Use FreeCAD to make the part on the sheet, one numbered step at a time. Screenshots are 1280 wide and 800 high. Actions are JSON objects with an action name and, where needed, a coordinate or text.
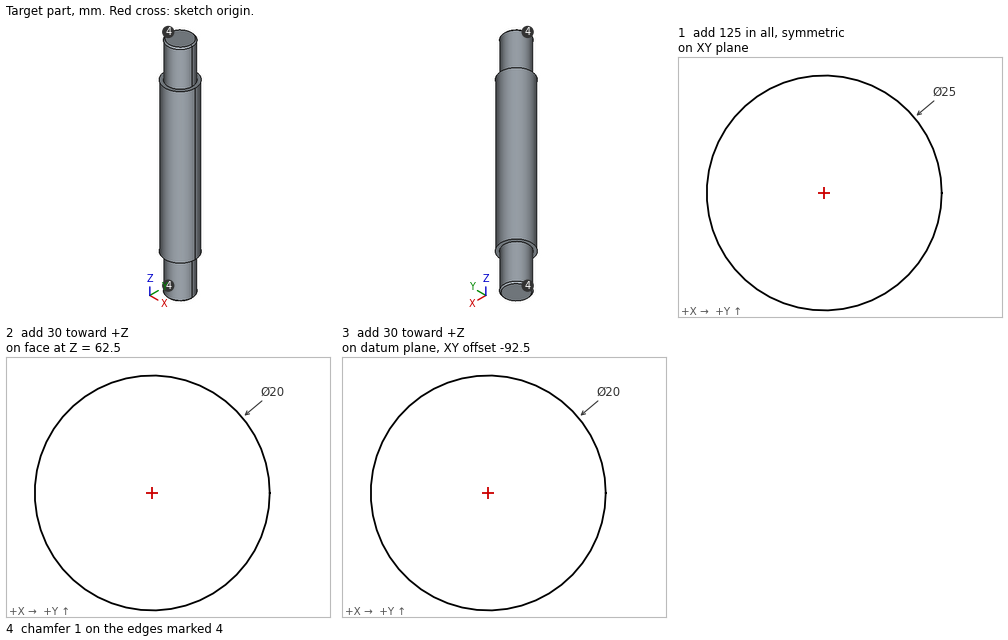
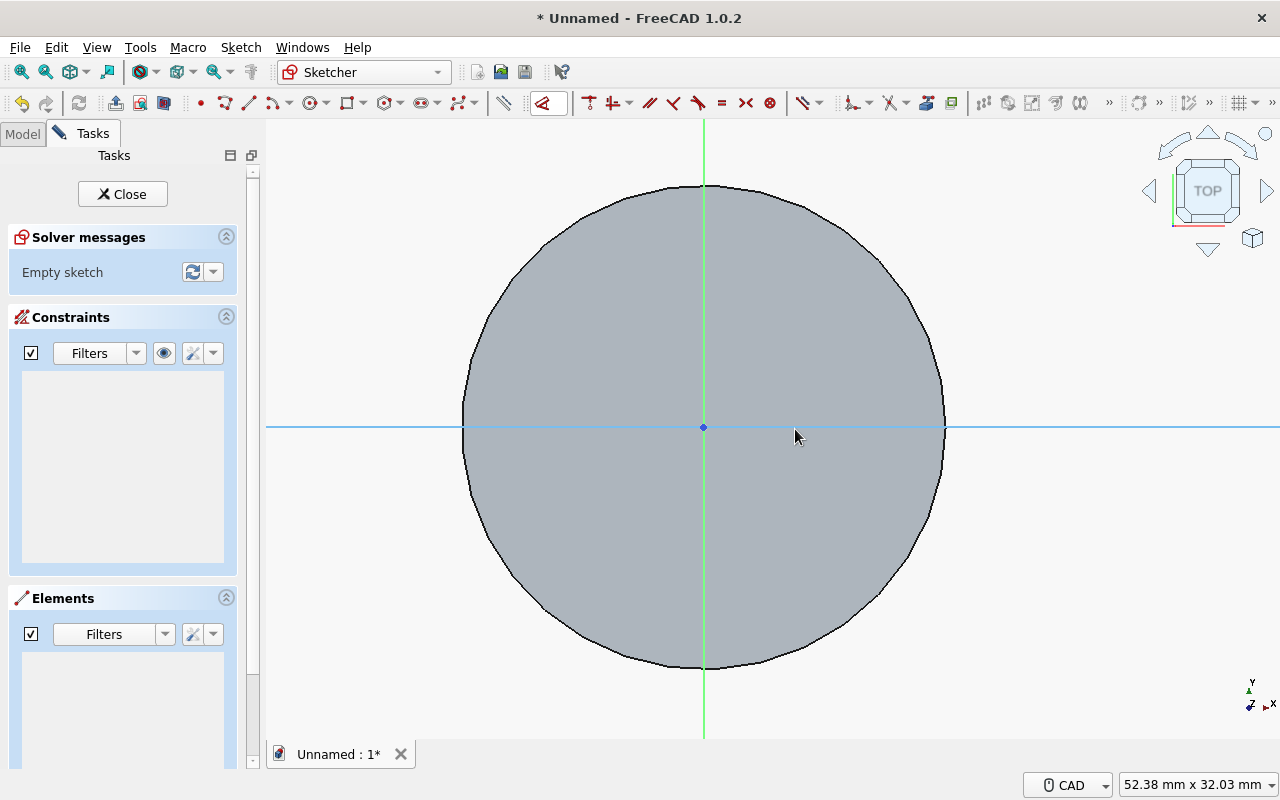
{"action": "left_click", "coordinate": [310, 104]}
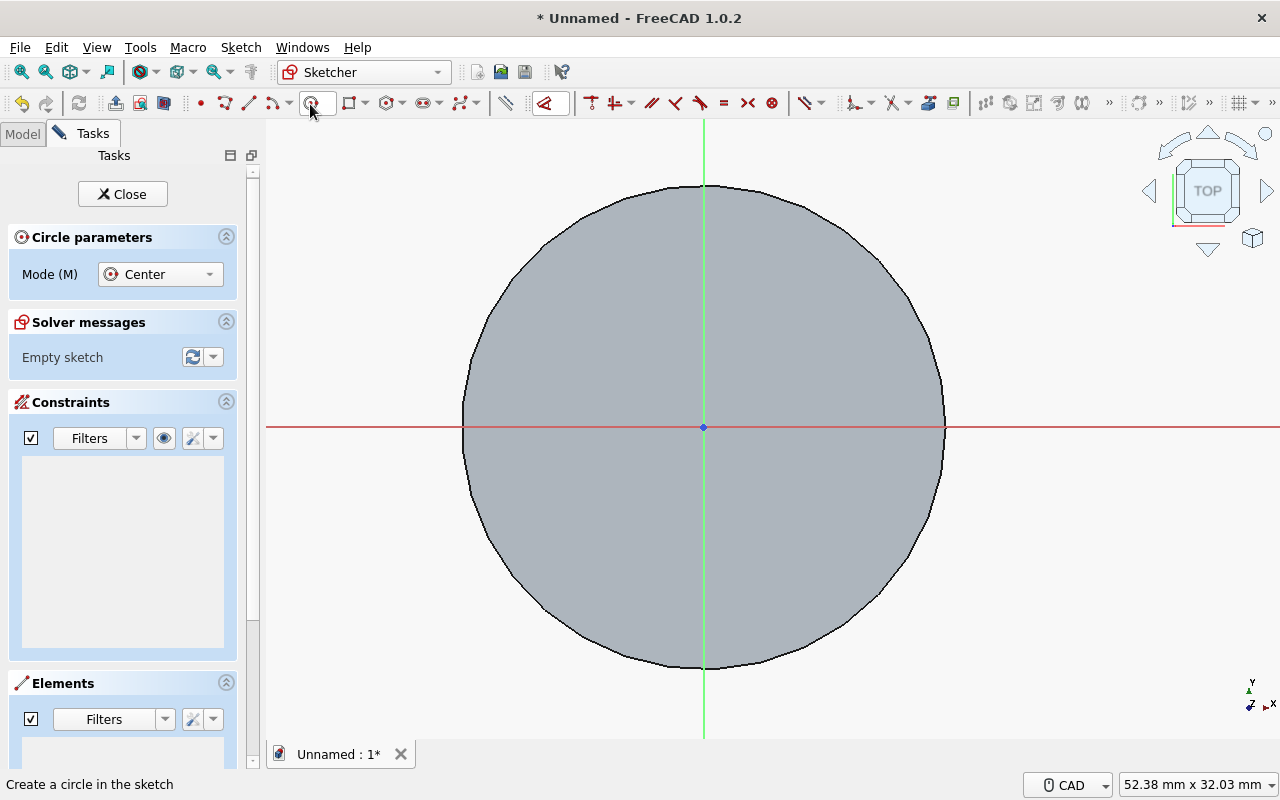
{"action": "left_click", "coordinate": [704, 427]}
{"action": "left_click", "coordinate": [841, 291]}
{"action": "key", "text": "Escape"}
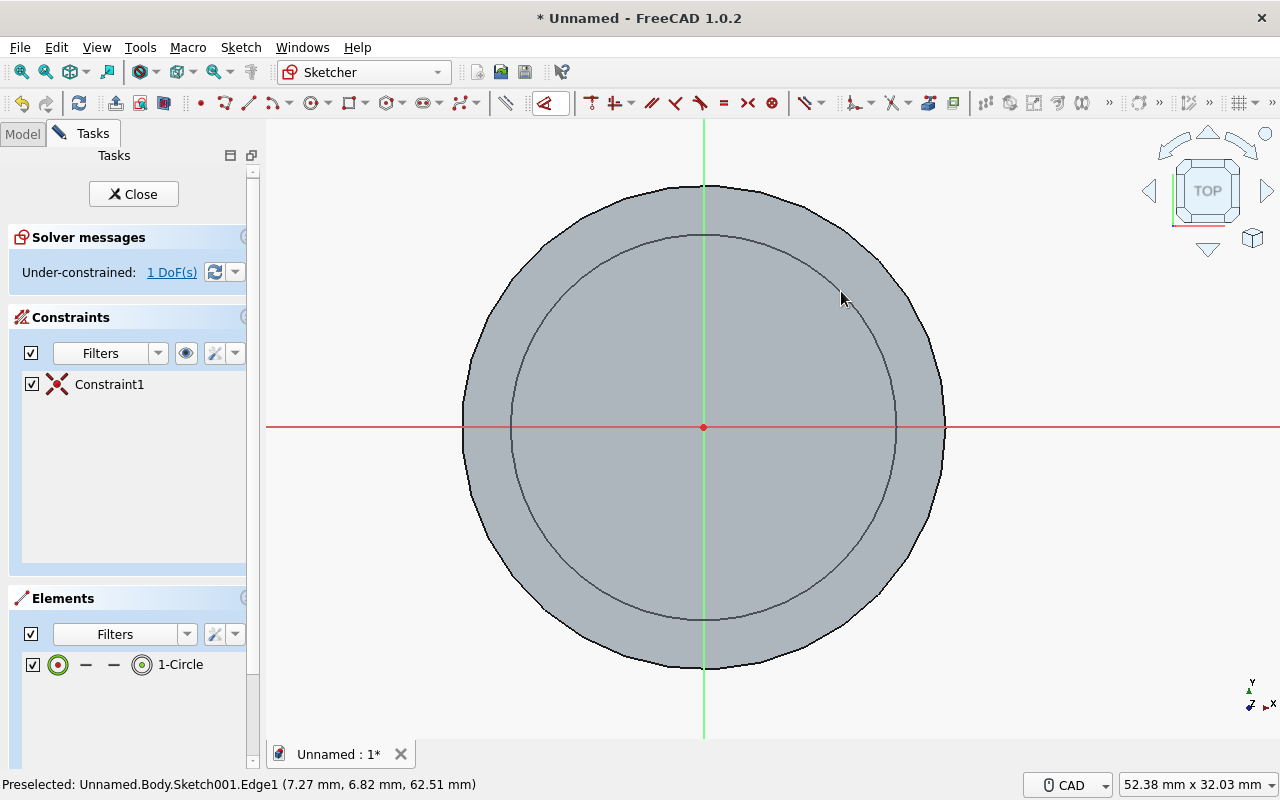
{"action": "left_click", "coordinate": [840, 291]}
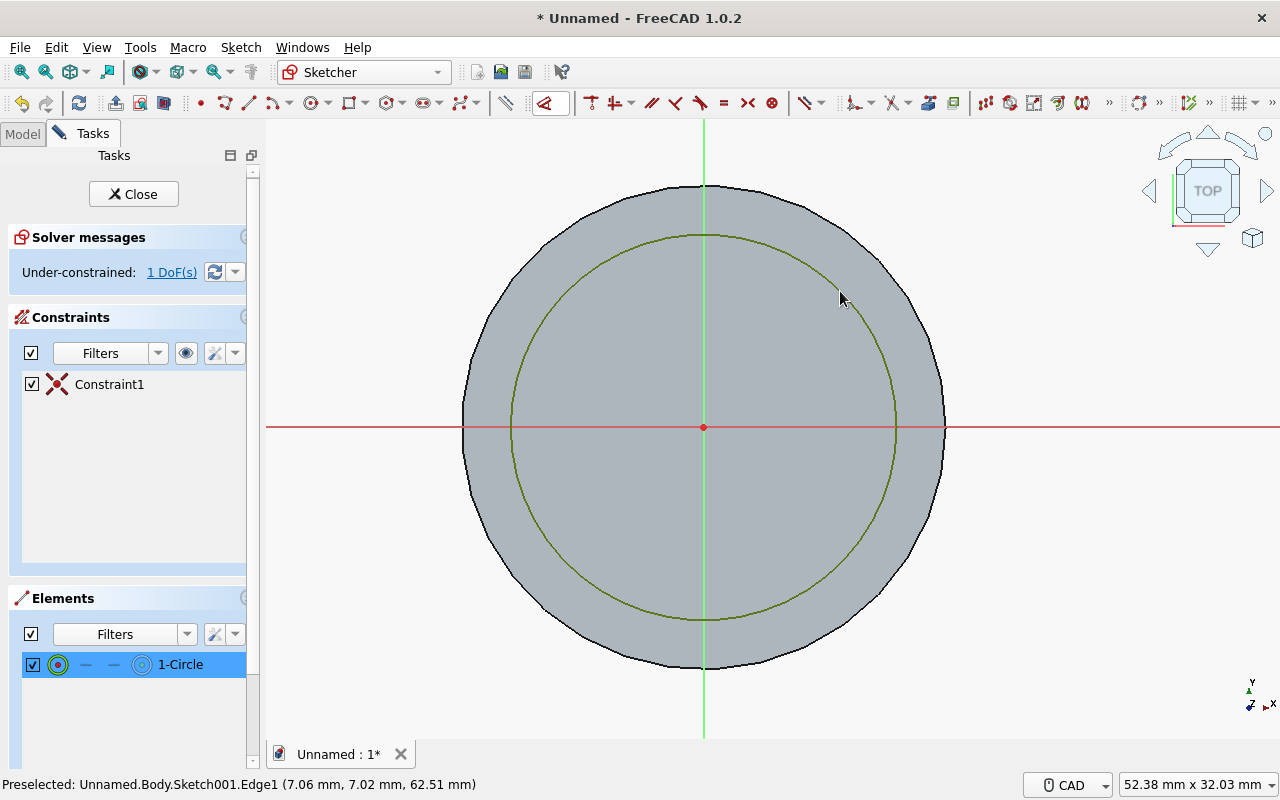
{"action": "left_click", "coordinate": [564, 104]}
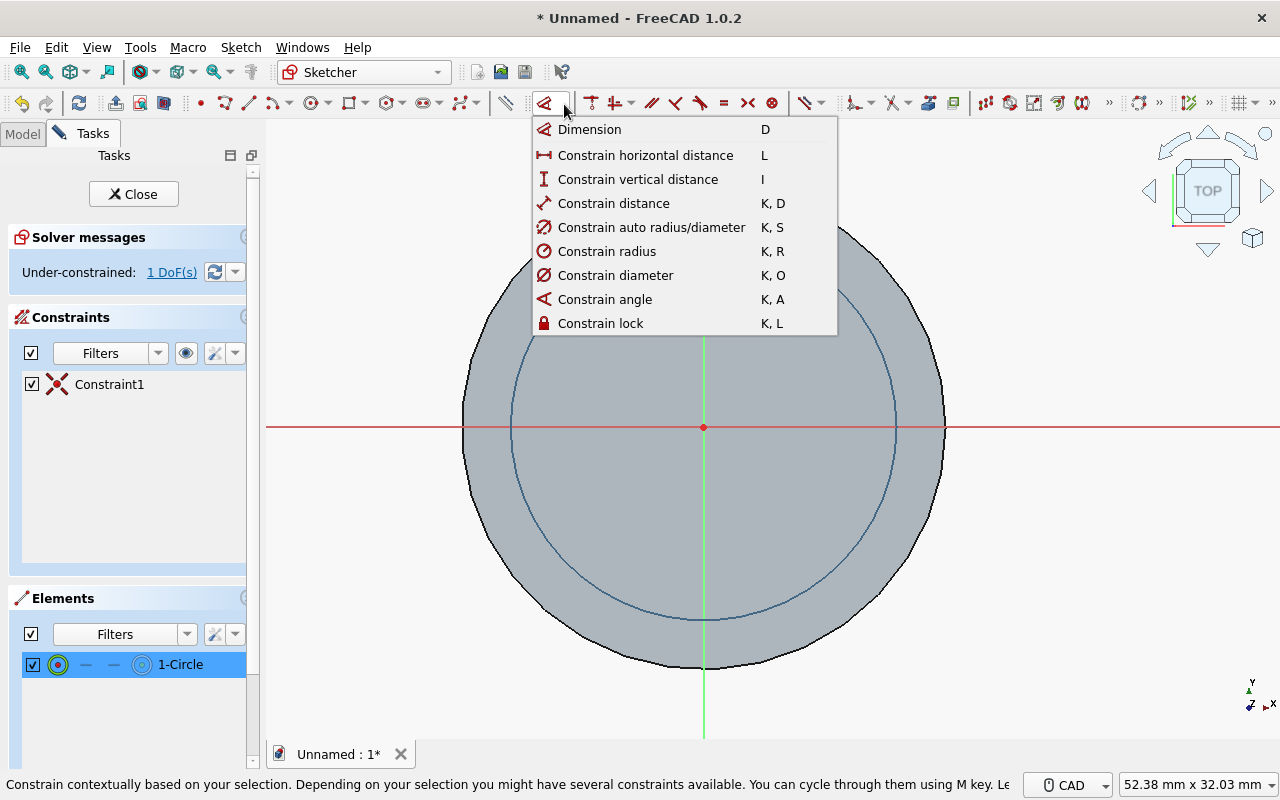
{"action": "left_click", "coordinate": [685, 275]}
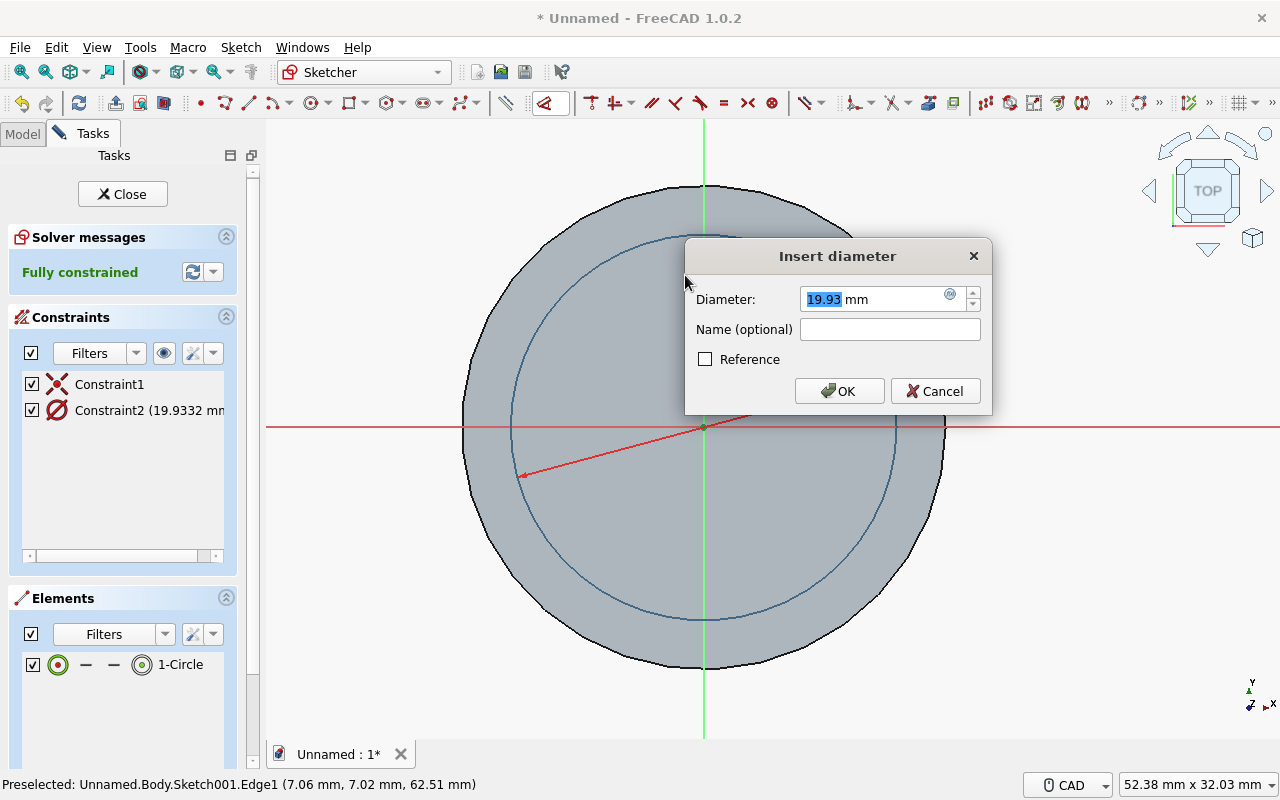
{"action": "type", "text": "20"}
{"action": "key", "text": "Return"}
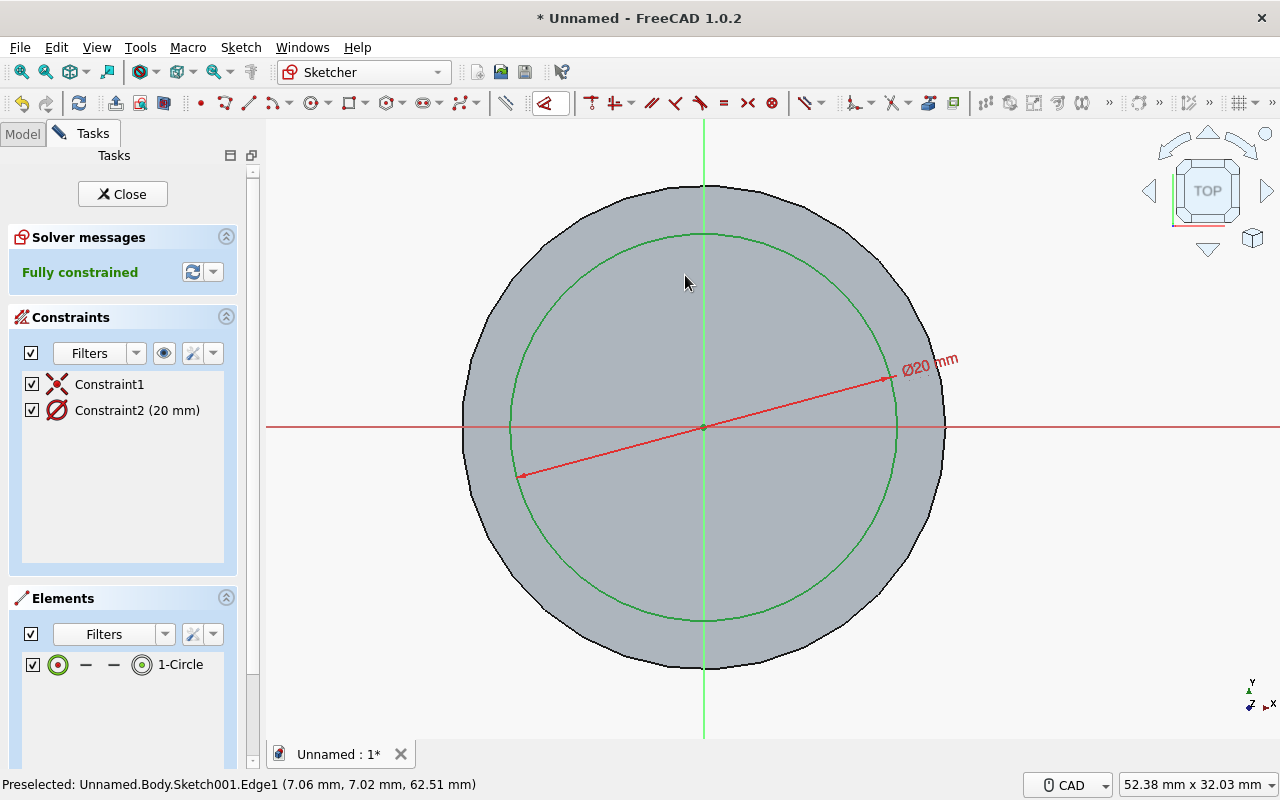
{"action": "left_click", "coordinate": [123, 194]}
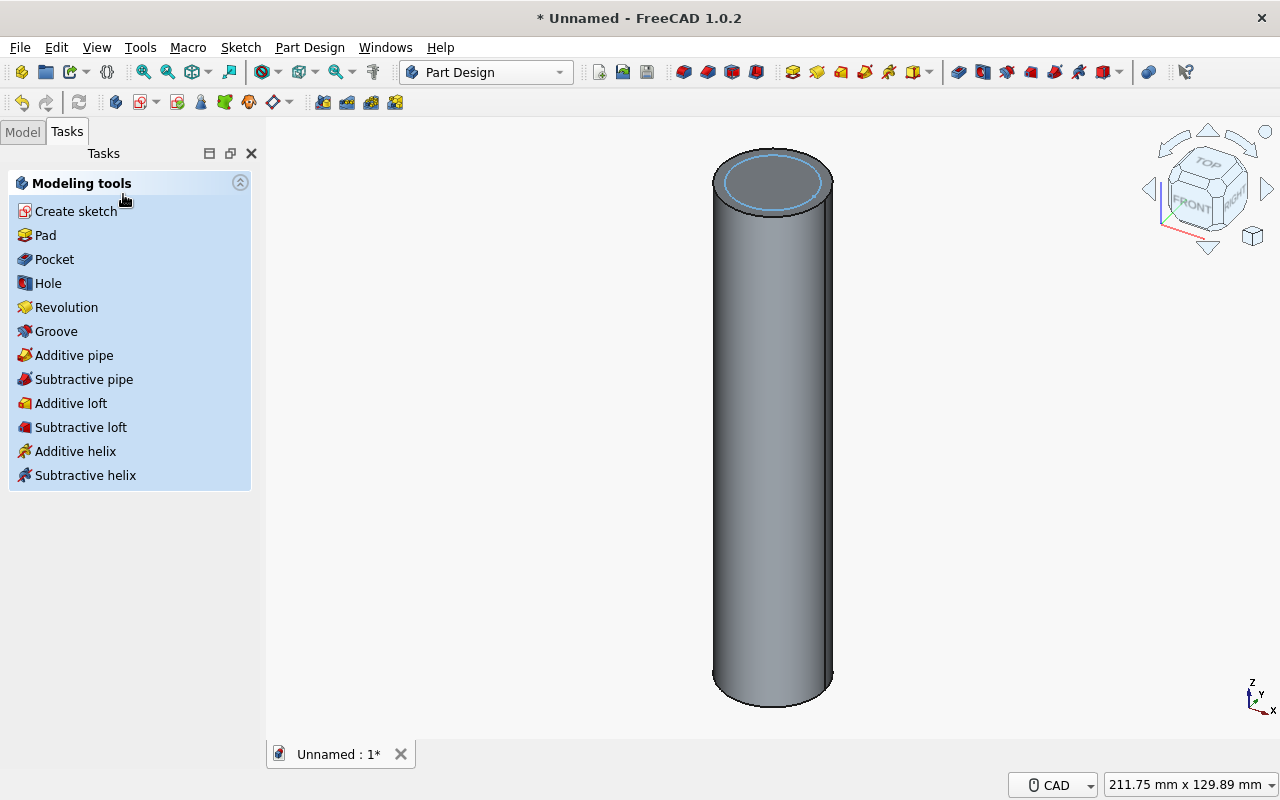
{"action": "left_click", "coordinate": [794, 72]}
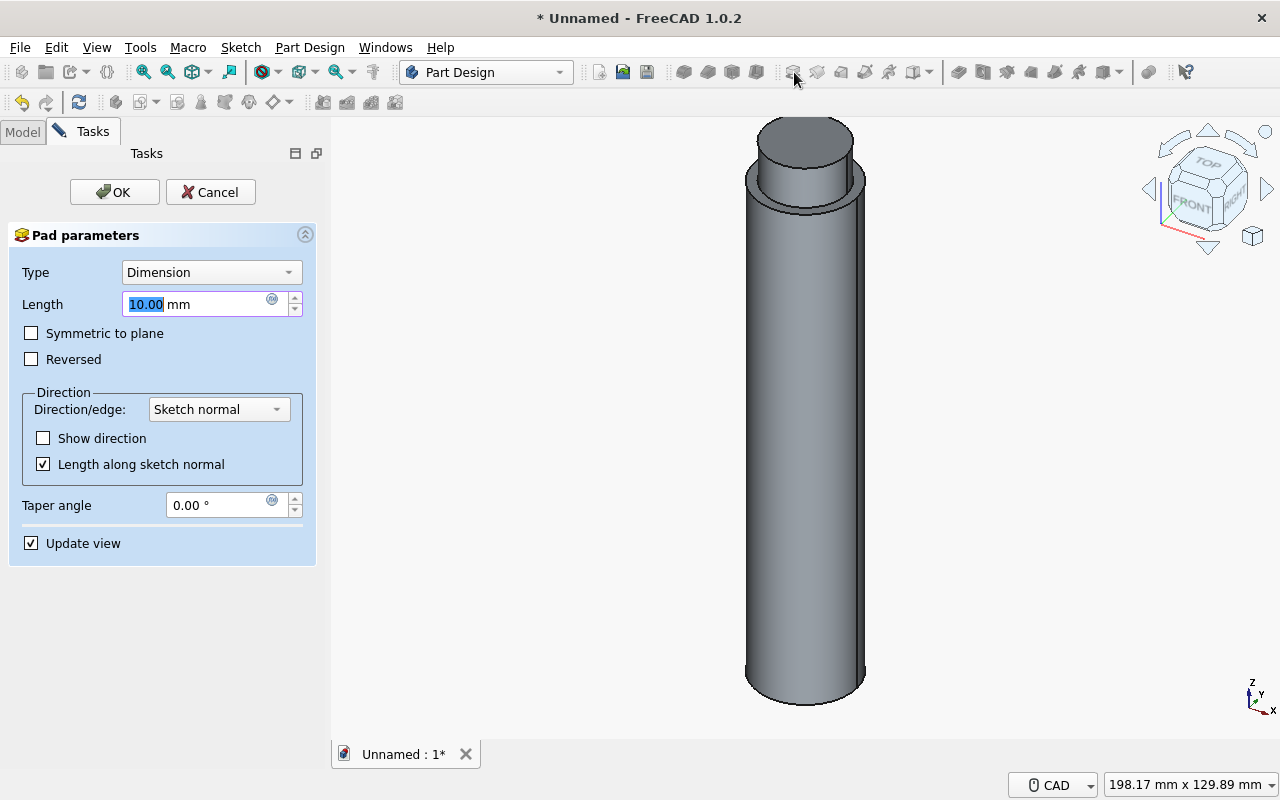
{"action": "type", "text": "30"}
{"action": "key", "text": "Tab"}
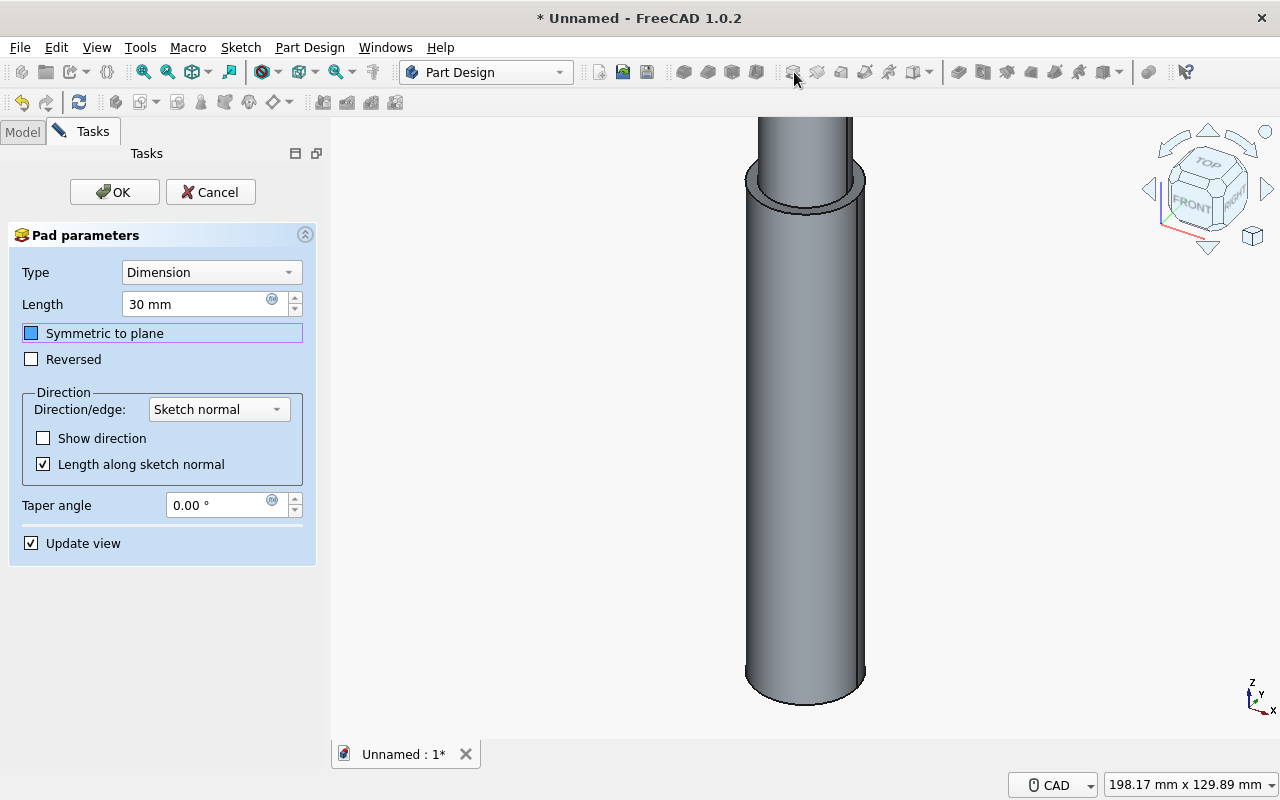
{"action": "left_click", "coordinate": [115, 192]}